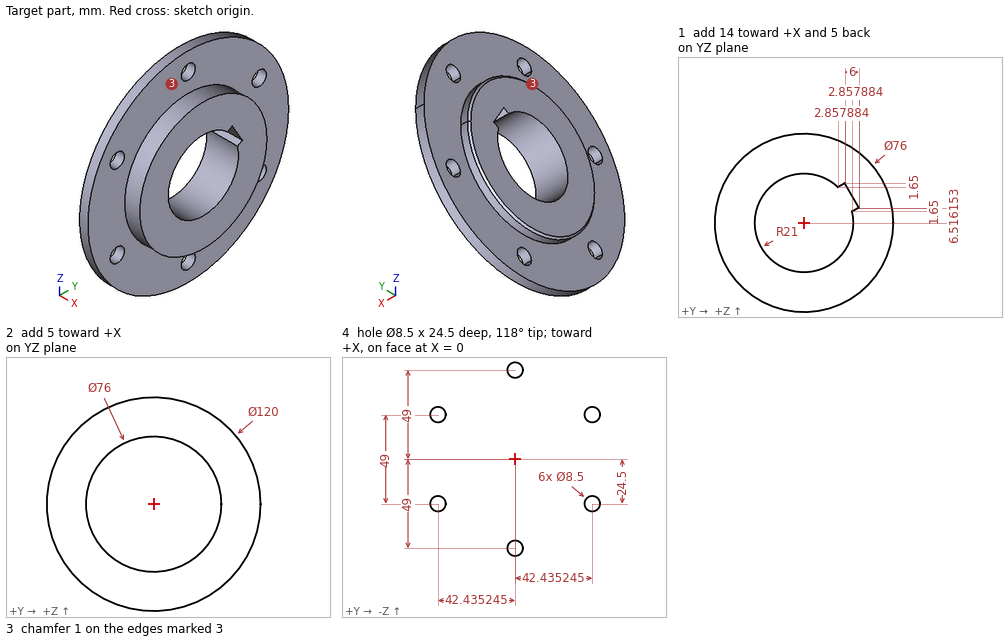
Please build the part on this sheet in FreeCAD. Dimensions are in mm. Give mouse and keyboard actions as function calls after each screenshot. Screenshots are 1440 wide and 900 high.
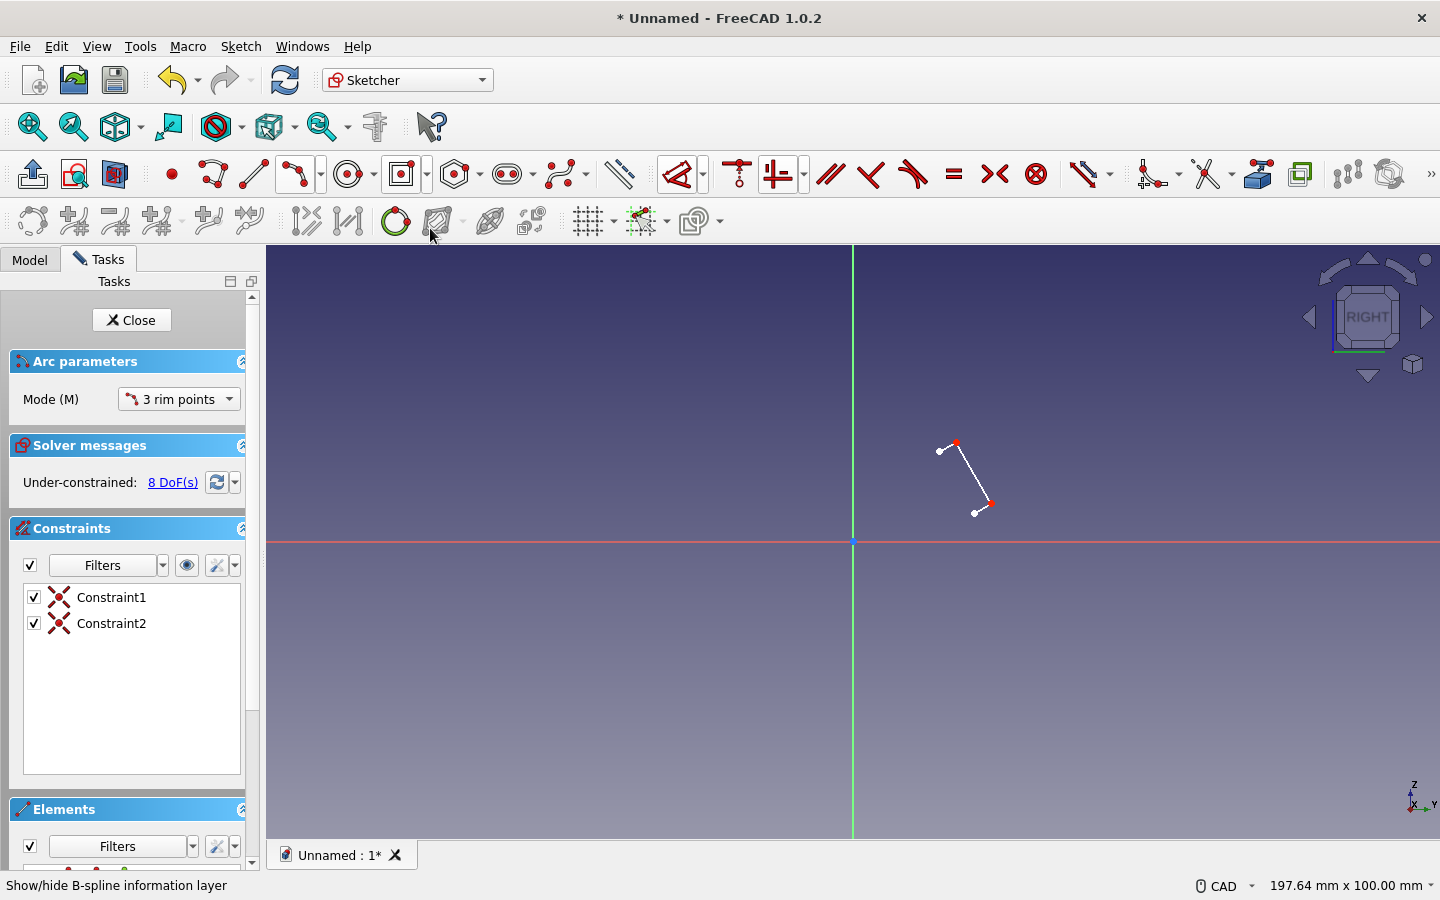
scroll(974, 513, up, 3)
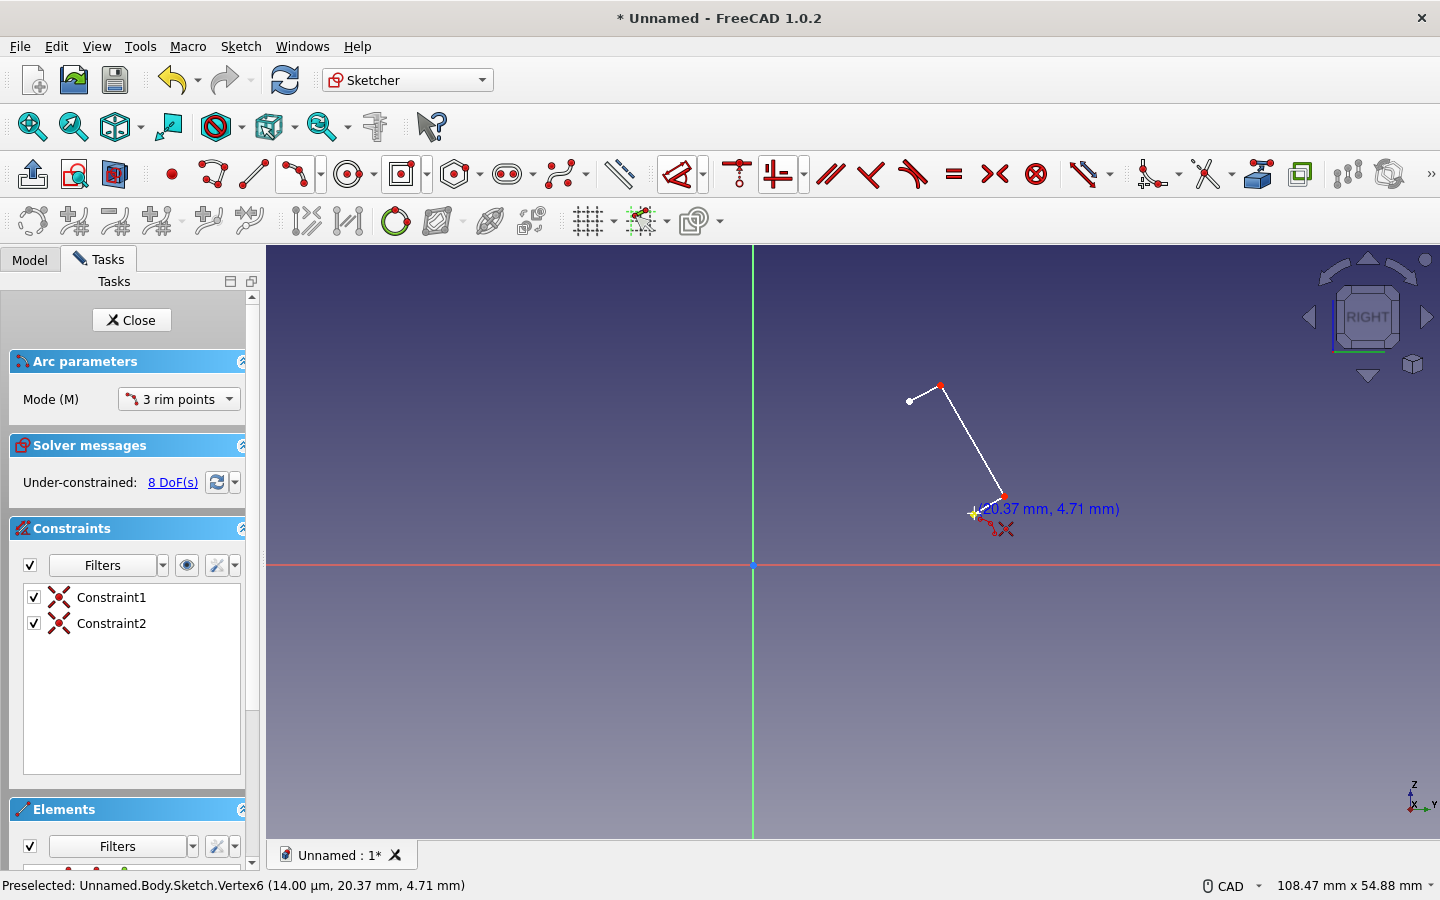
click(974, 514)
click(910, 401)
click(556, 679)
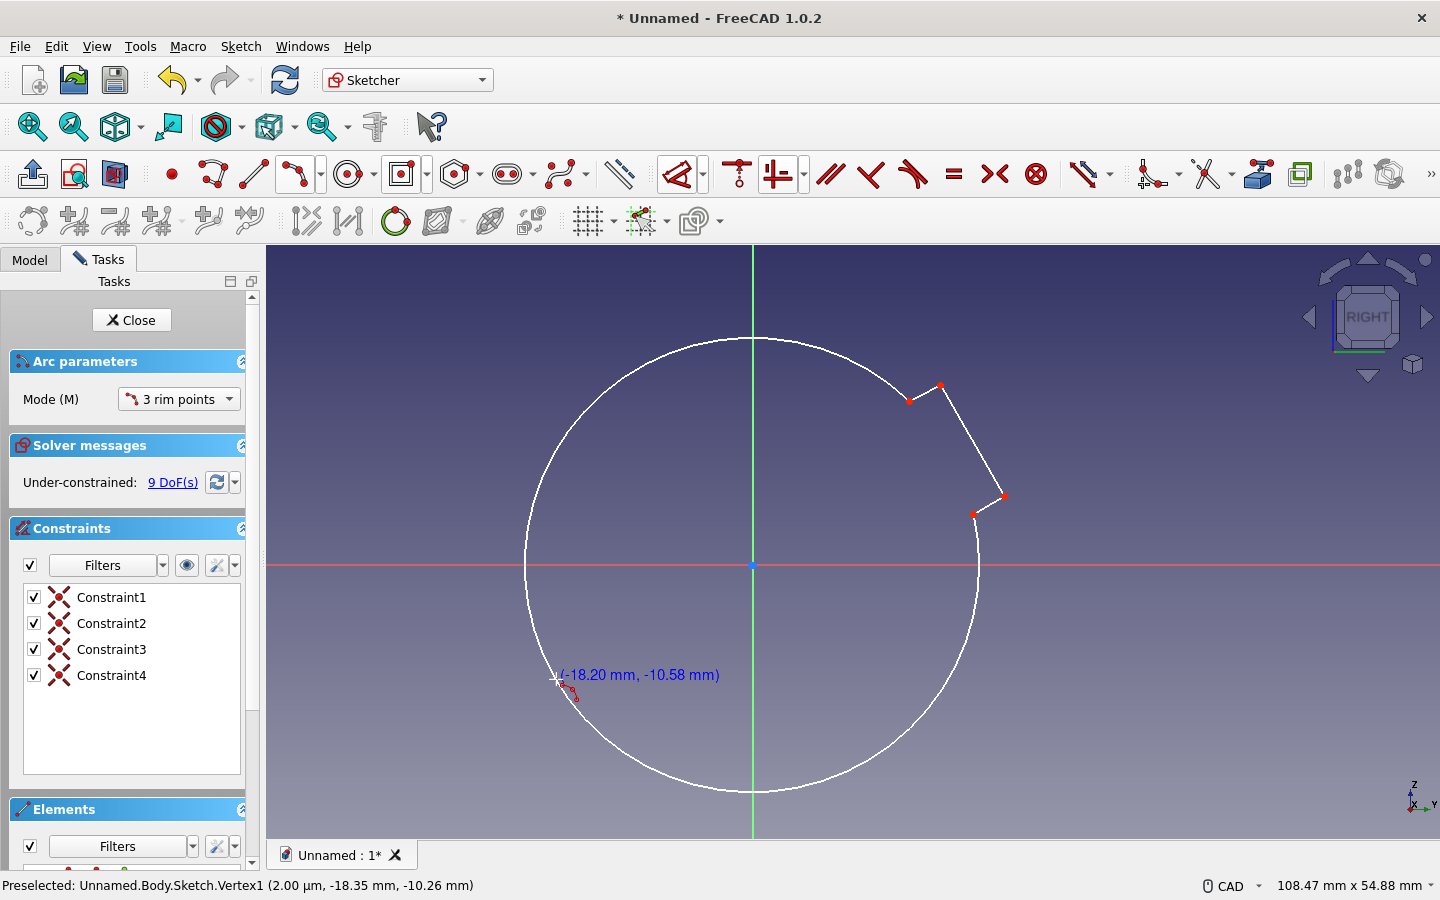
key(g)
key(c)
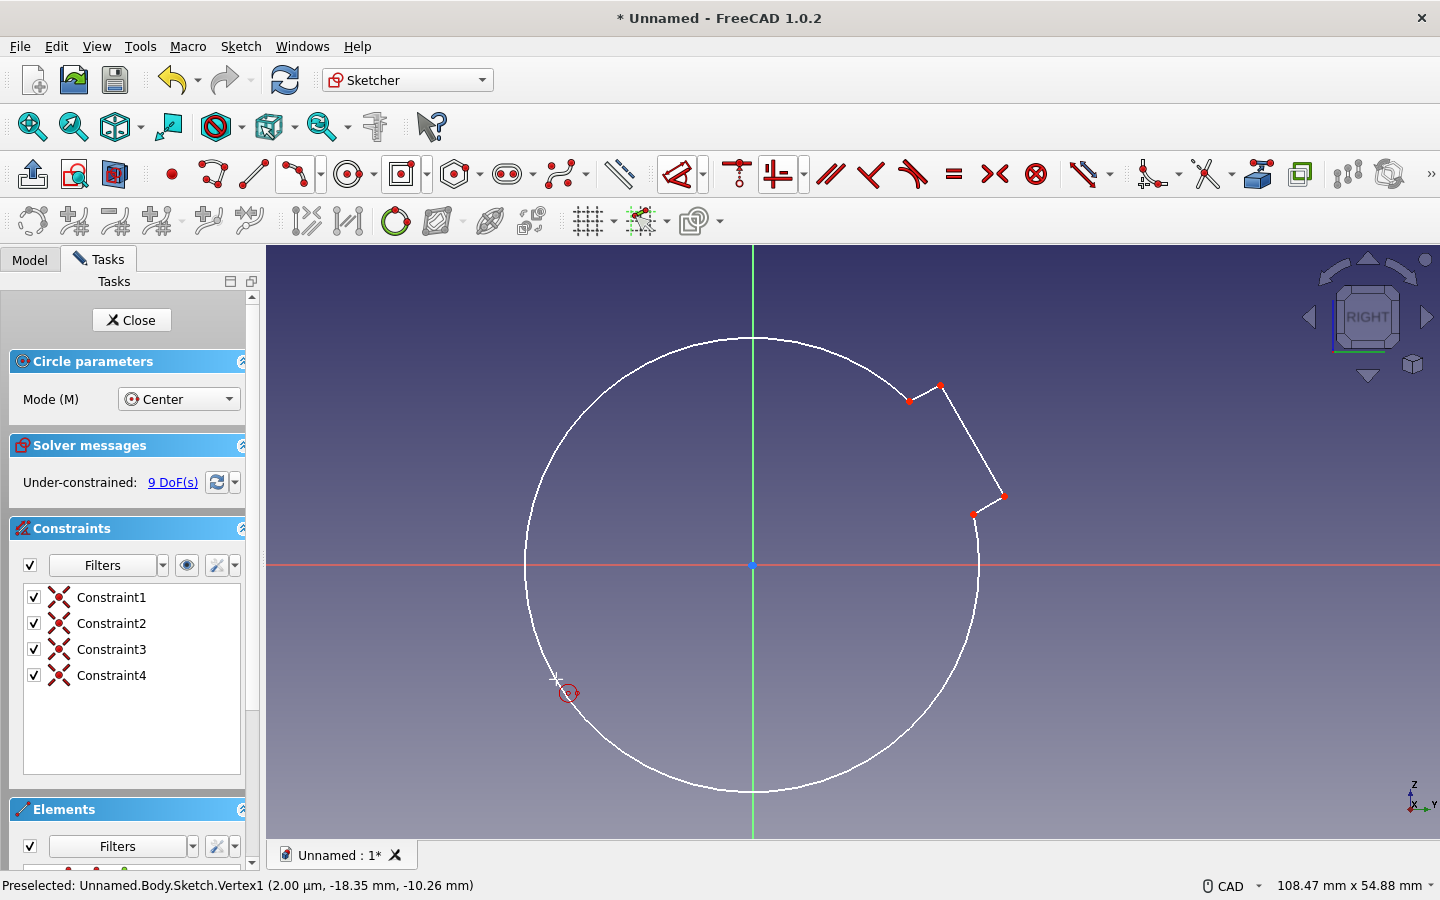
click(753, 565)
move(1044, 275)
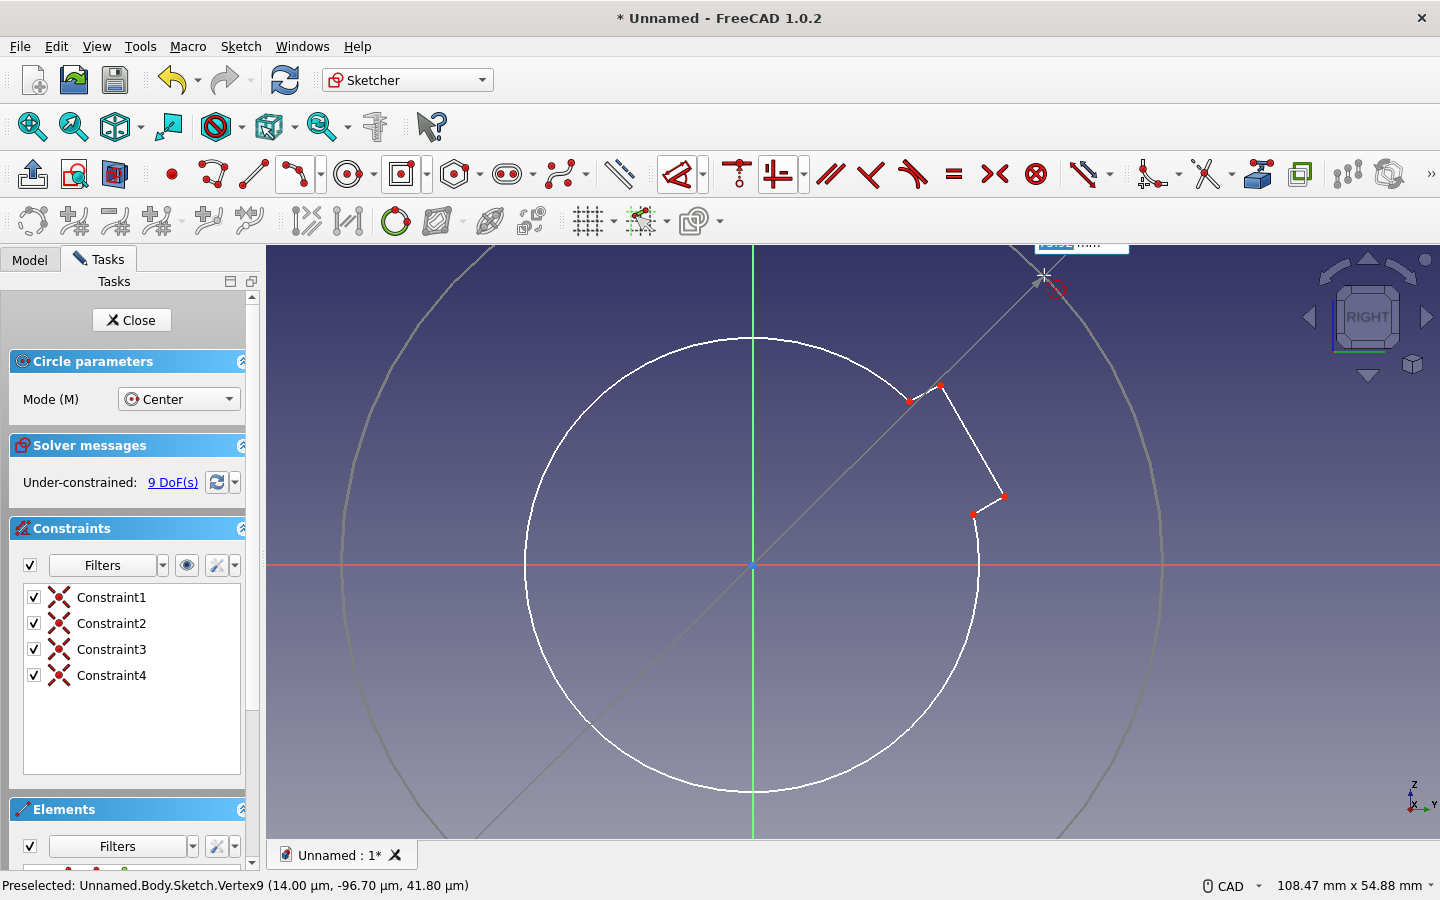
text(76)
key(Return)
key(Escape)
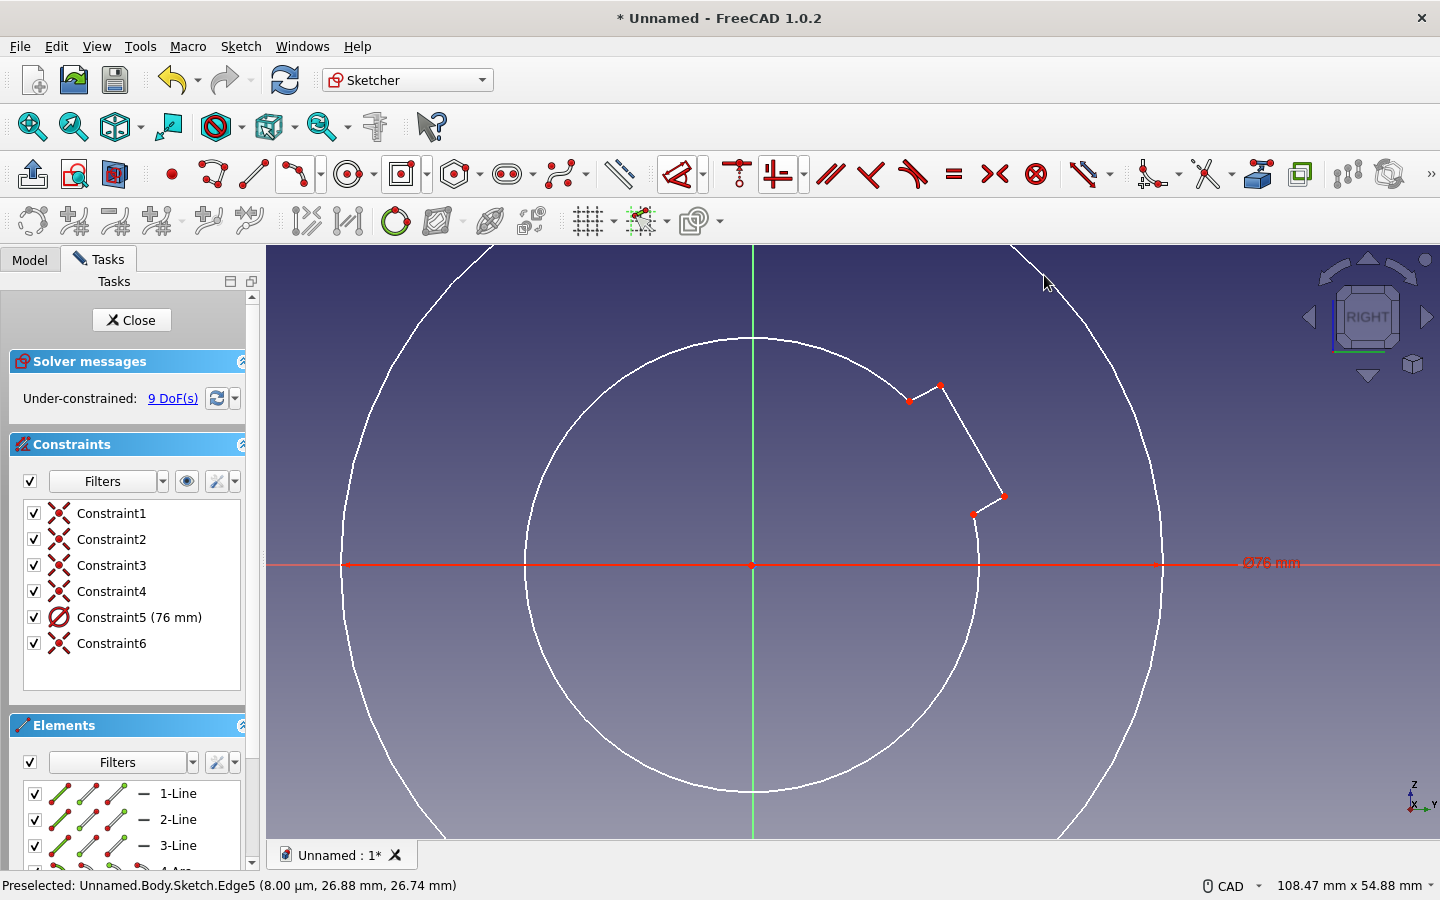
drag(742, 555, 763, 575)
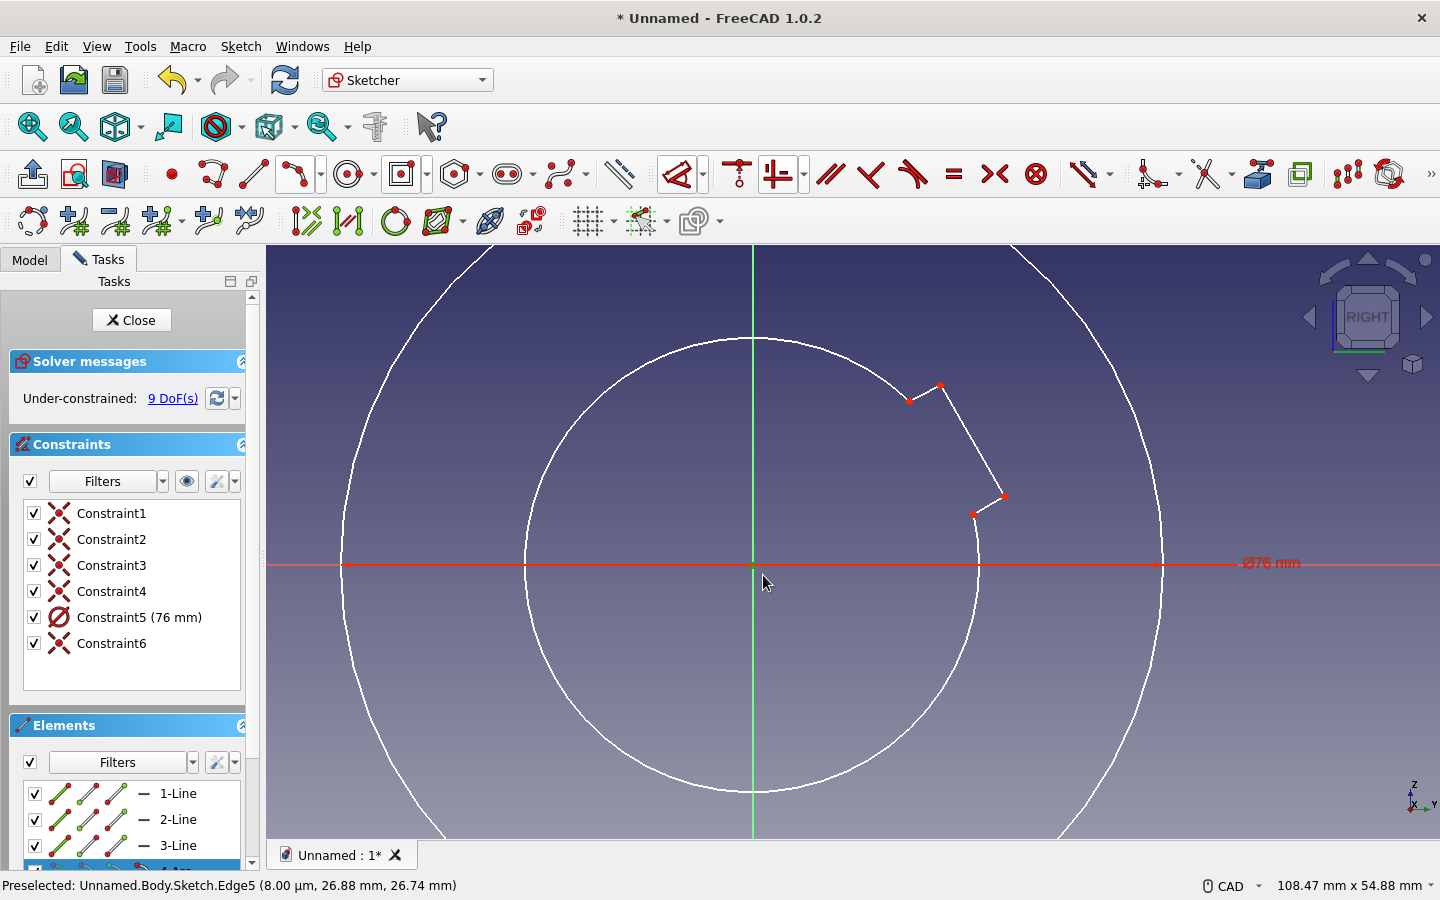
click(737, 174)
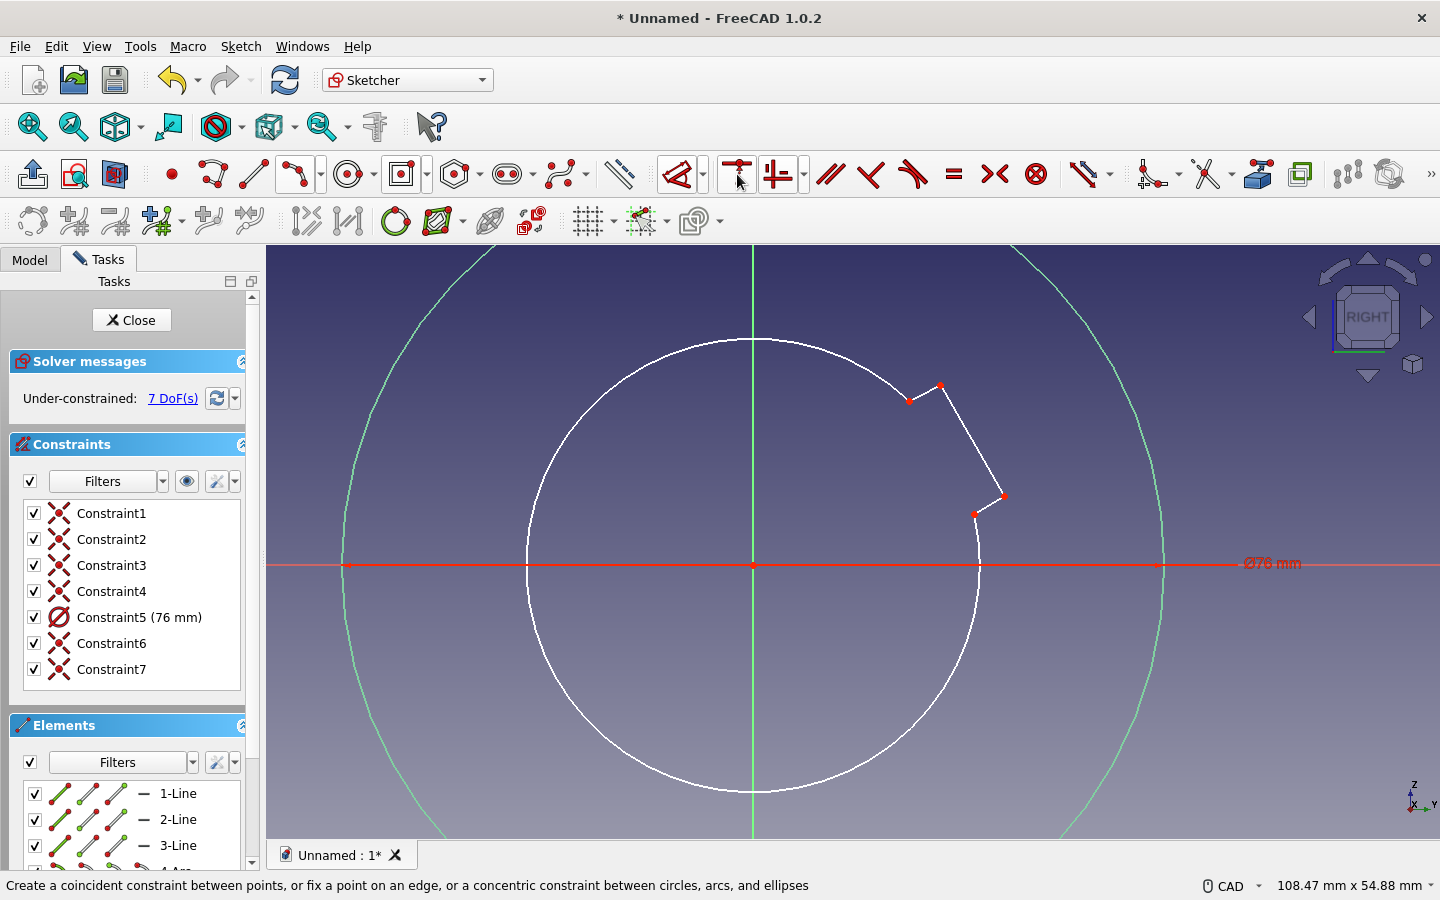
key(d)